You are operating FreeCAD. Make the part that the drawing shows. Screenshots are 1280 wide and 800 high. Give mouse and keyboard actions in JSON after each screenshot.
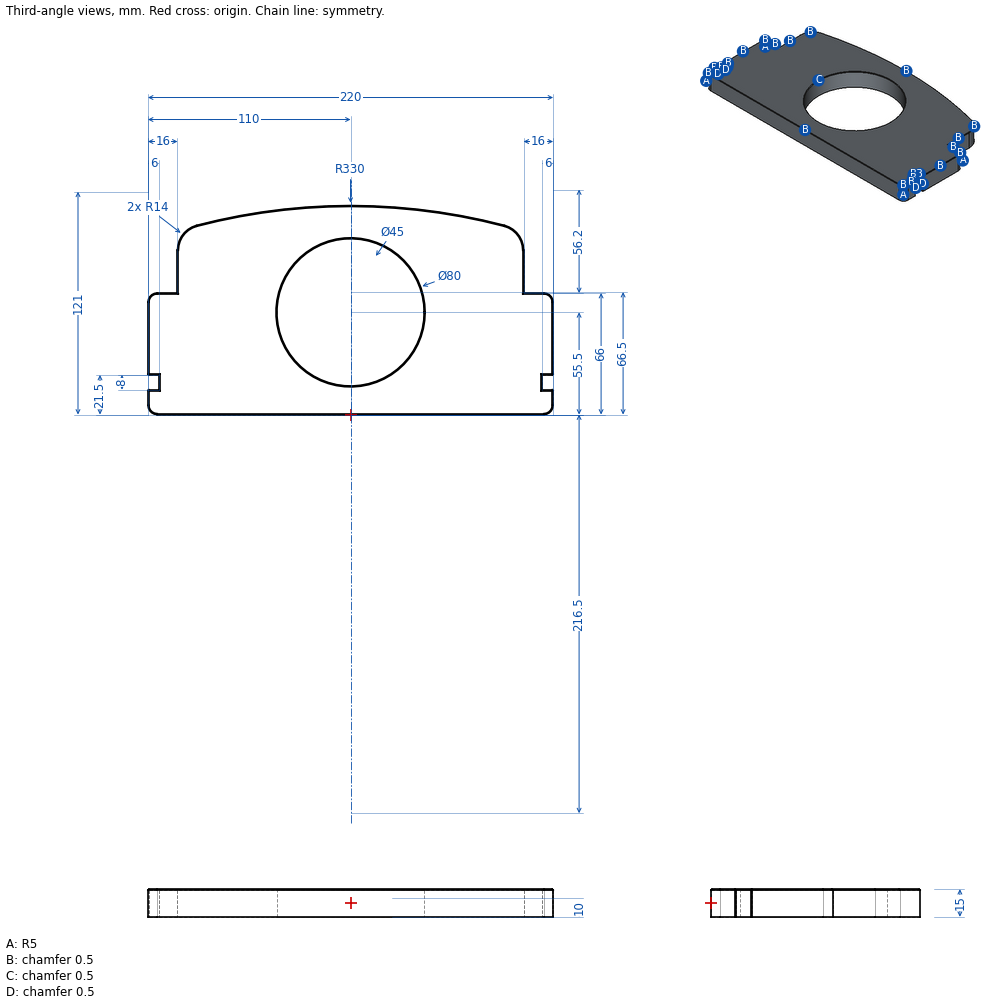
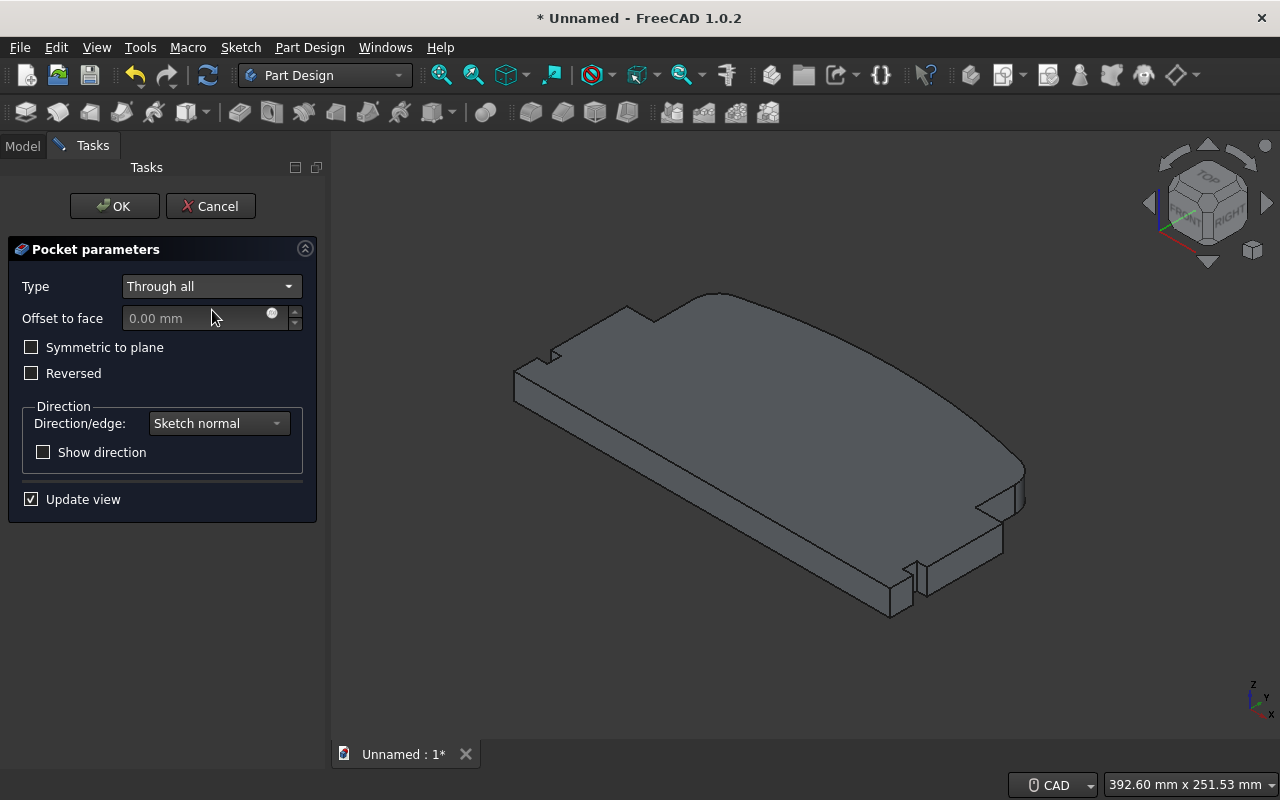
{"action": "left_click", "coordinate": [115, 206]}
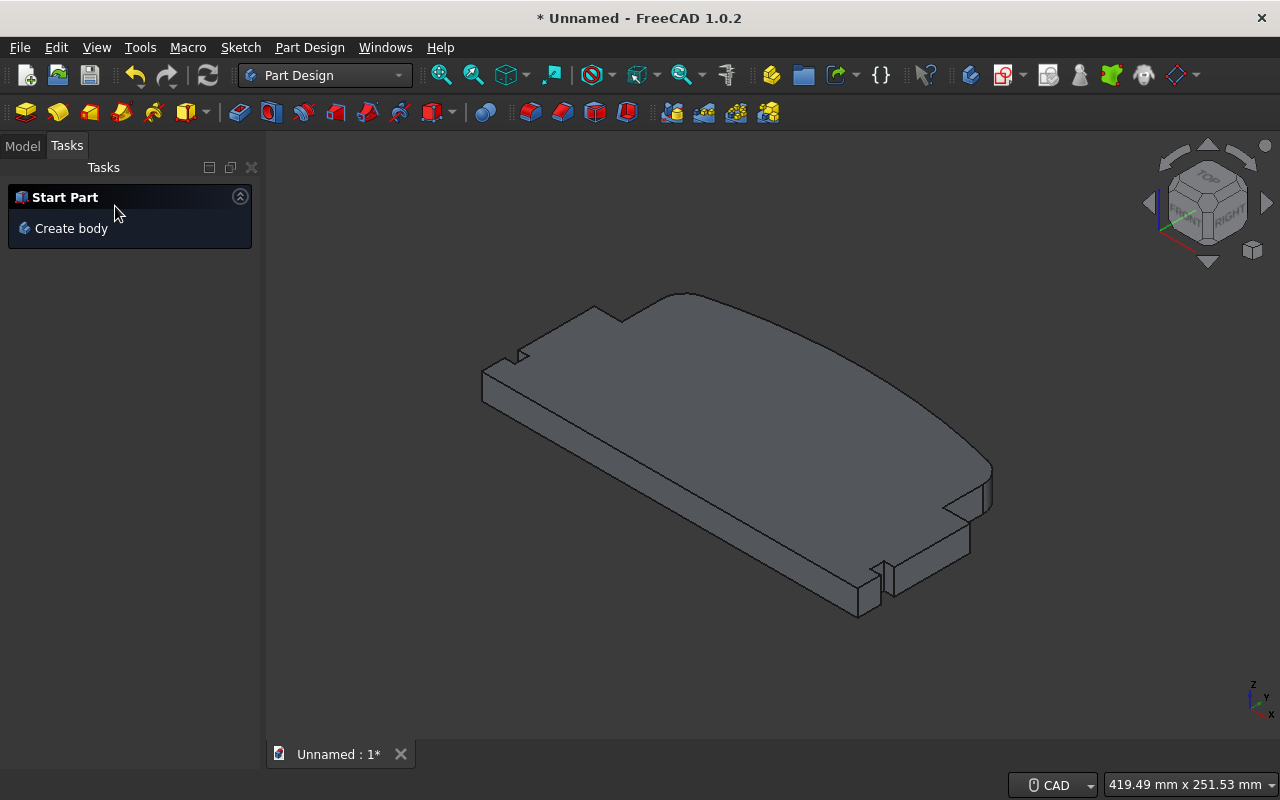
{"action": "left_click", "coordinate": [858, 602]}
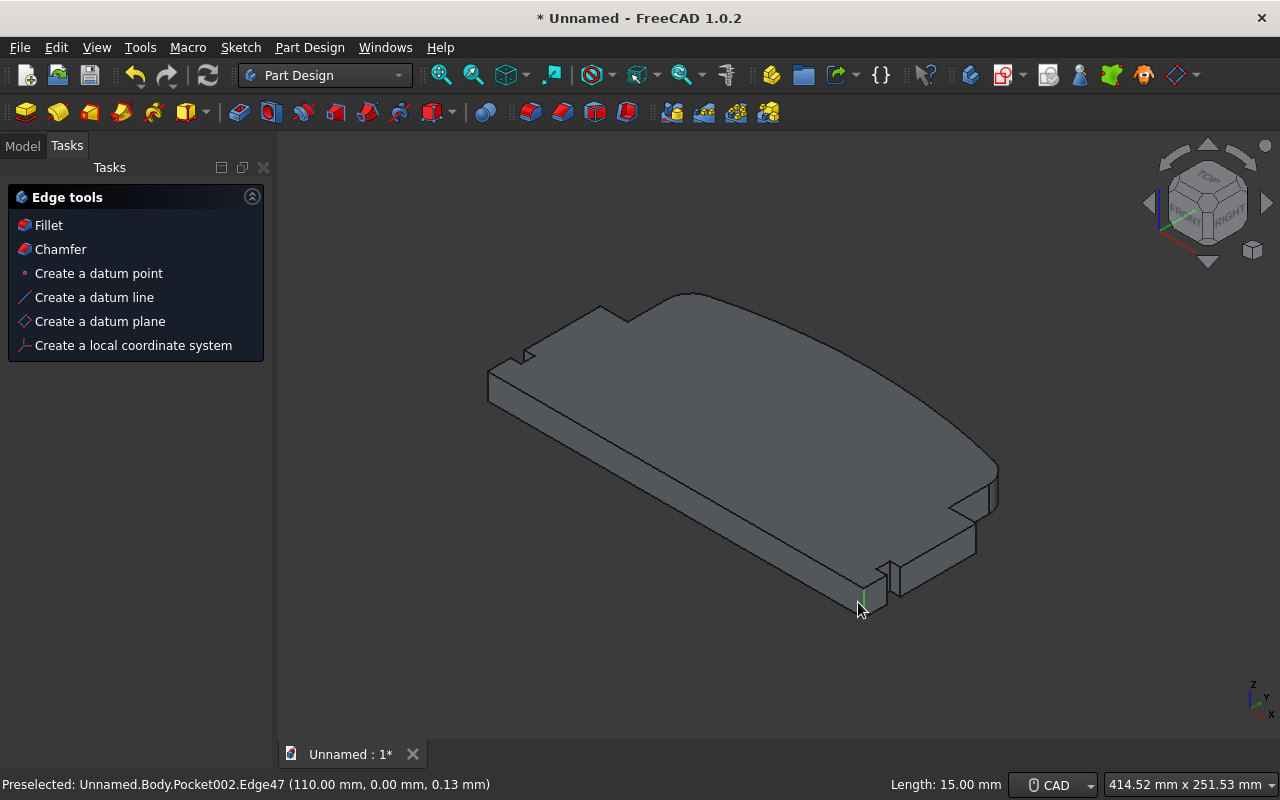
{"action": "key", "text": "2"}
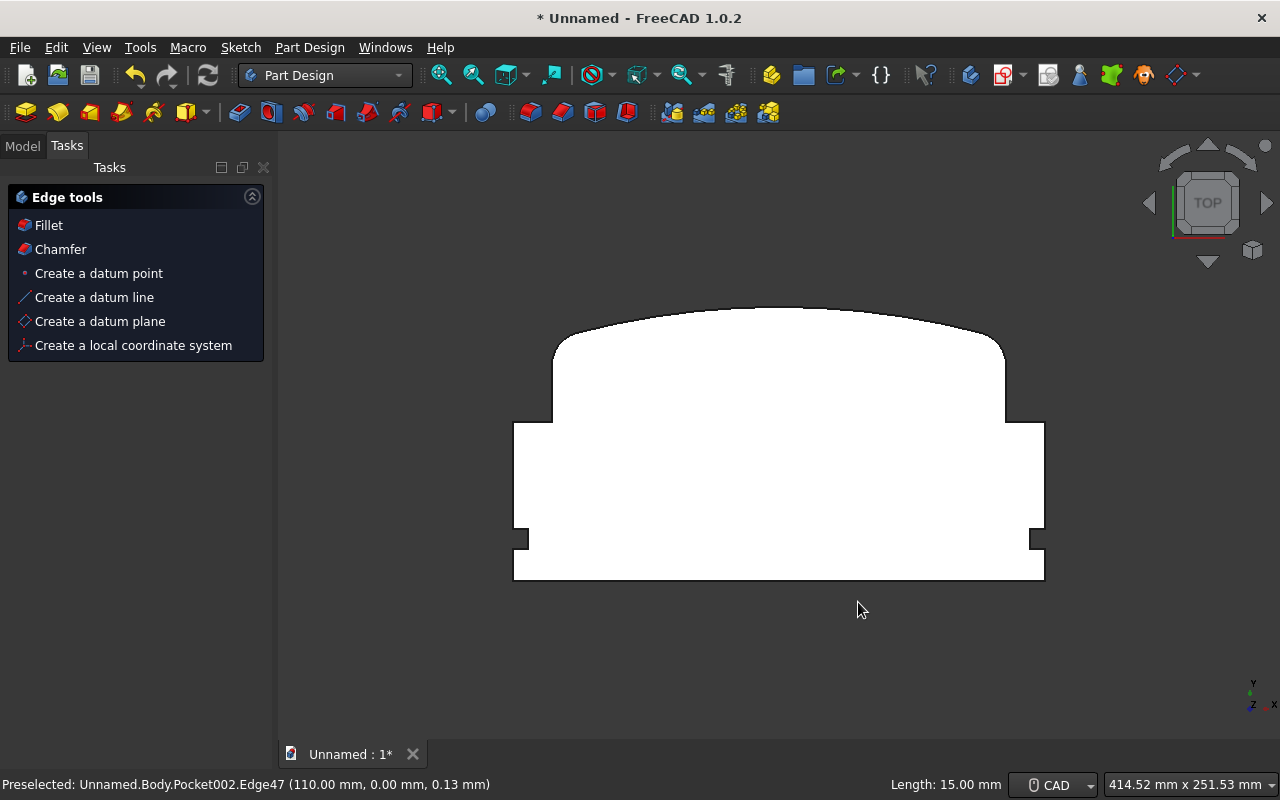
{"action": "key", "text": "0"}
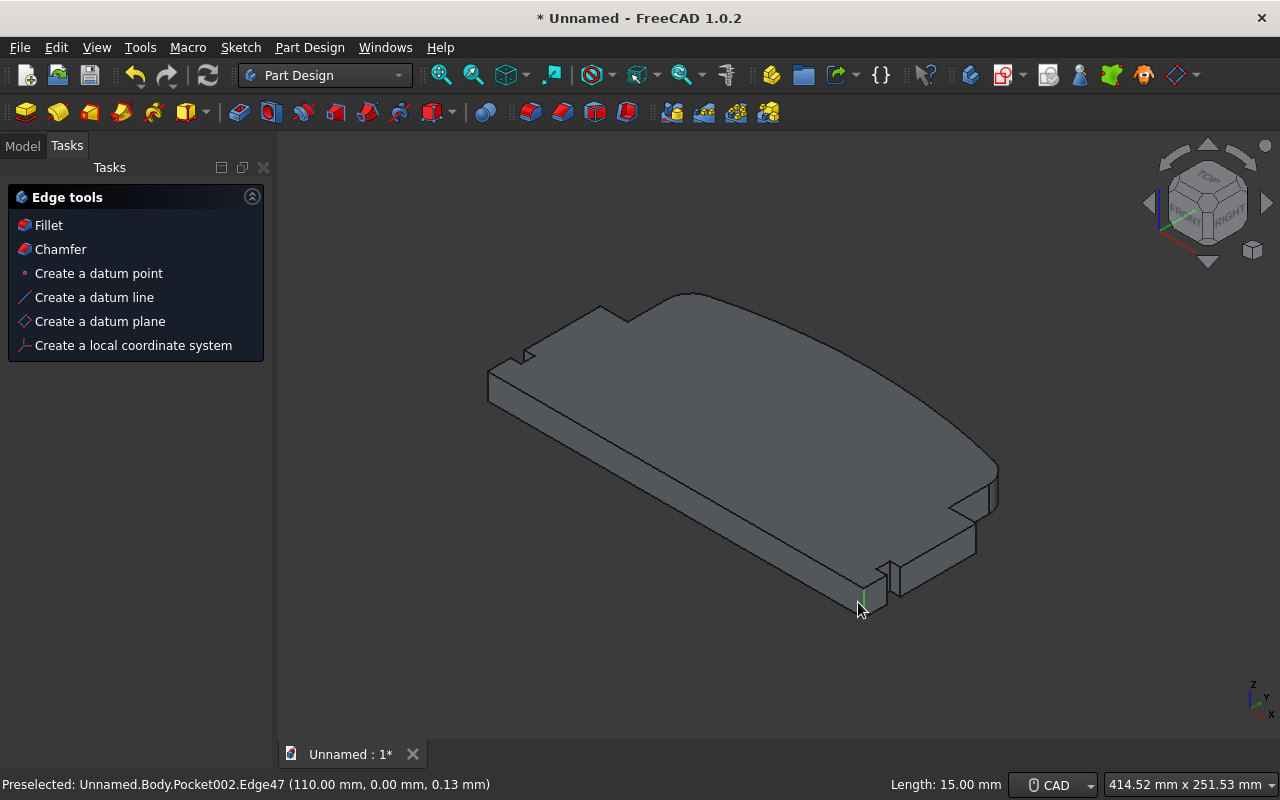
{"action": "key", "text": "1"}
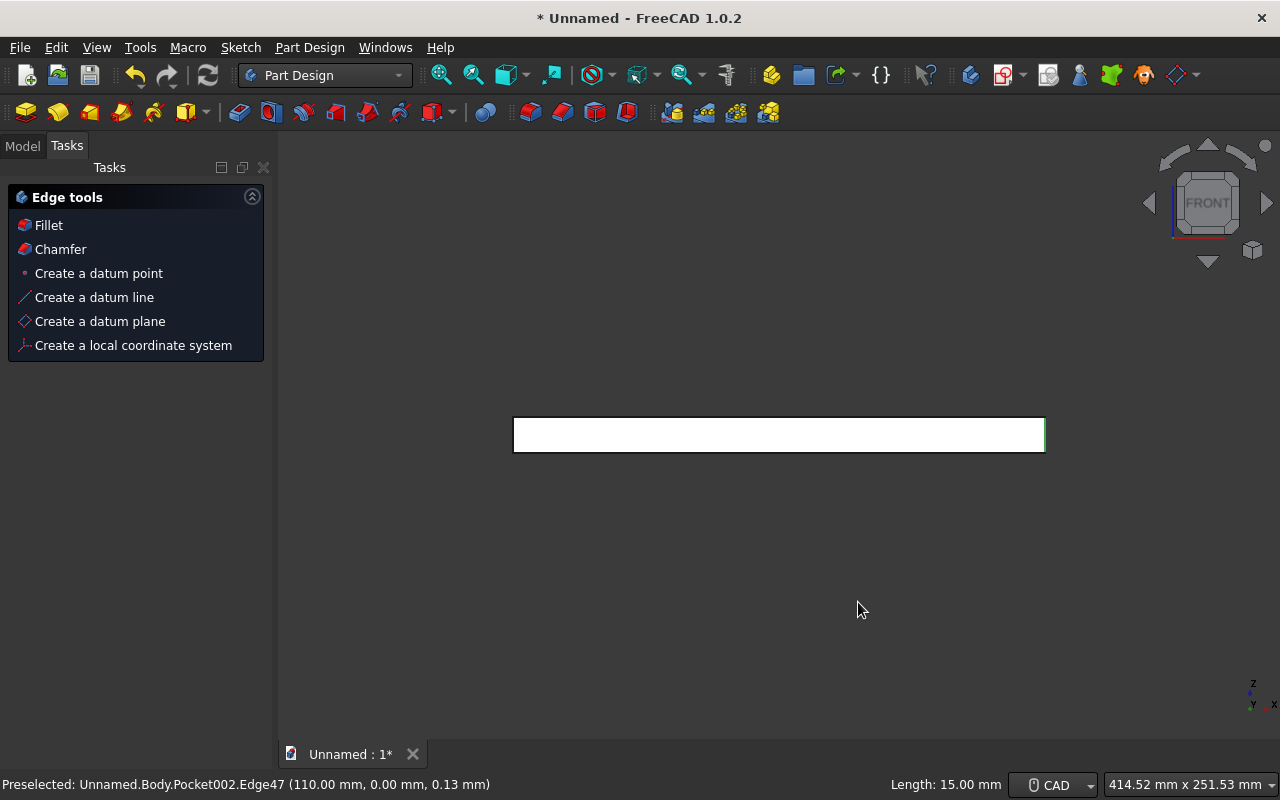
{"action": "left_click", "coordinate": [513, 434], "text": "ctrl"}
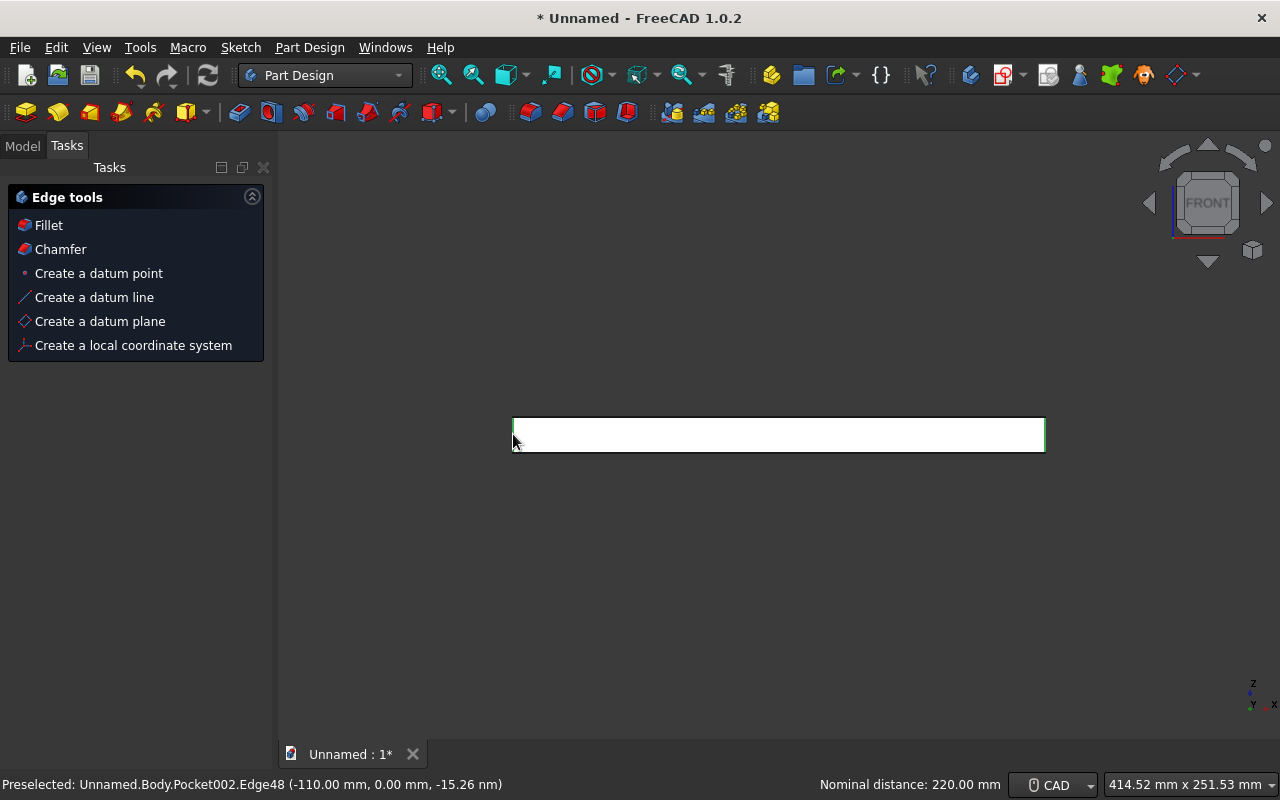
{"action": "key", "text": "3"}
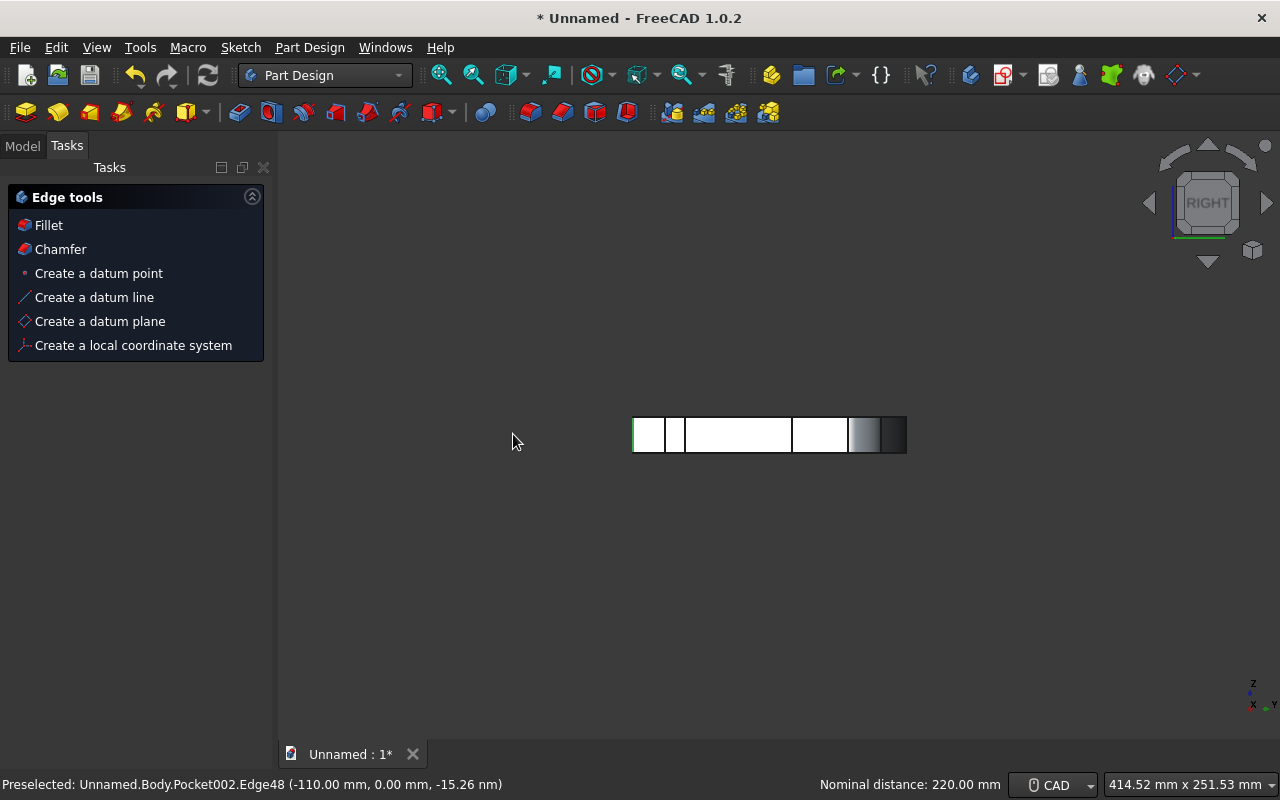
{"action": "left_click", "coordinate": [442, 76]}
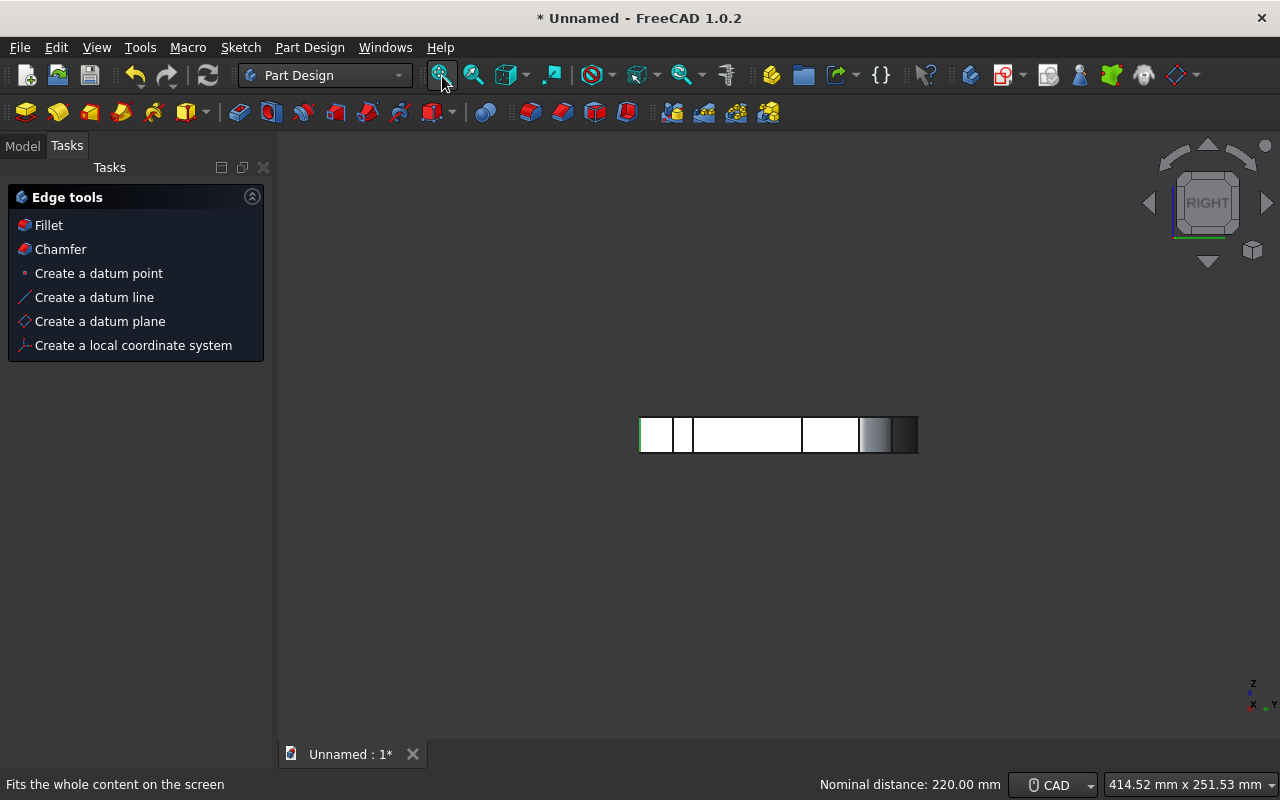
{"action": "left_click", "coordinate": [802, 434], "text": "ctrl"}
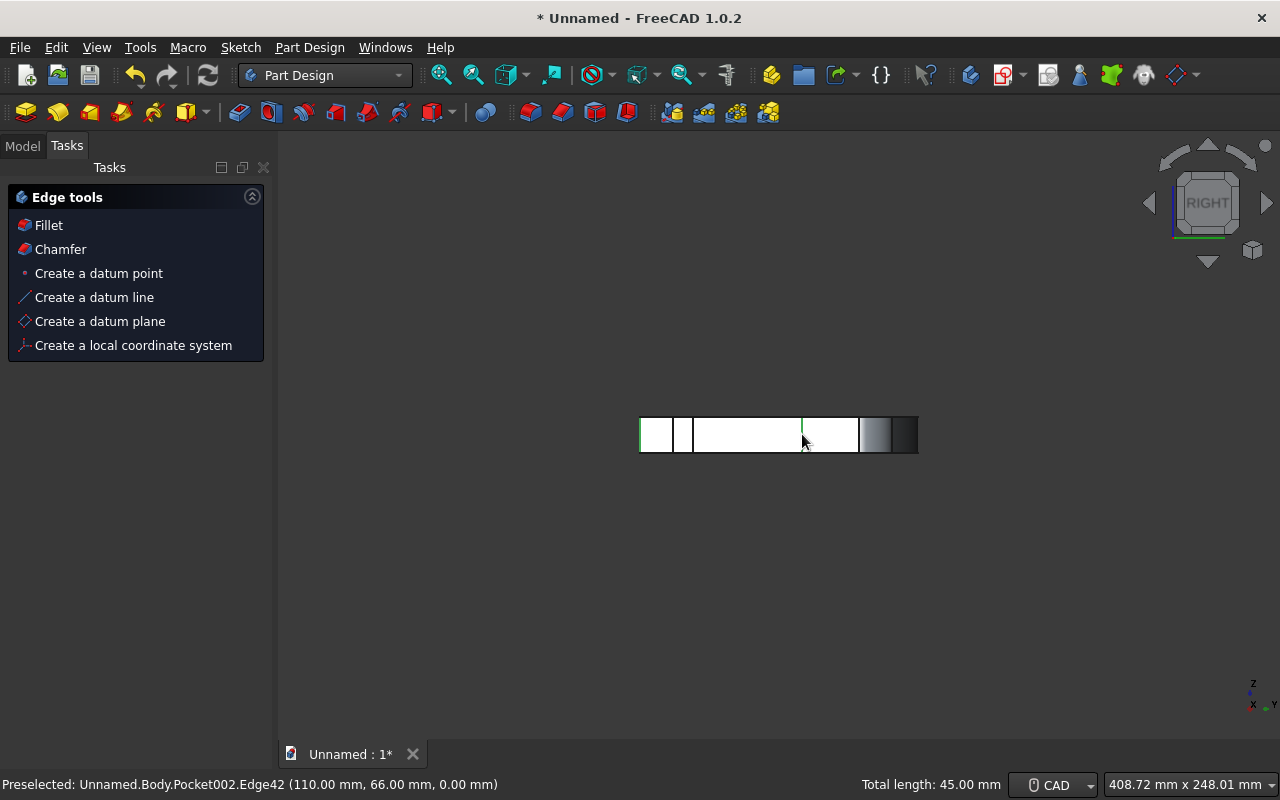
{"action": "key", "text": "5"}